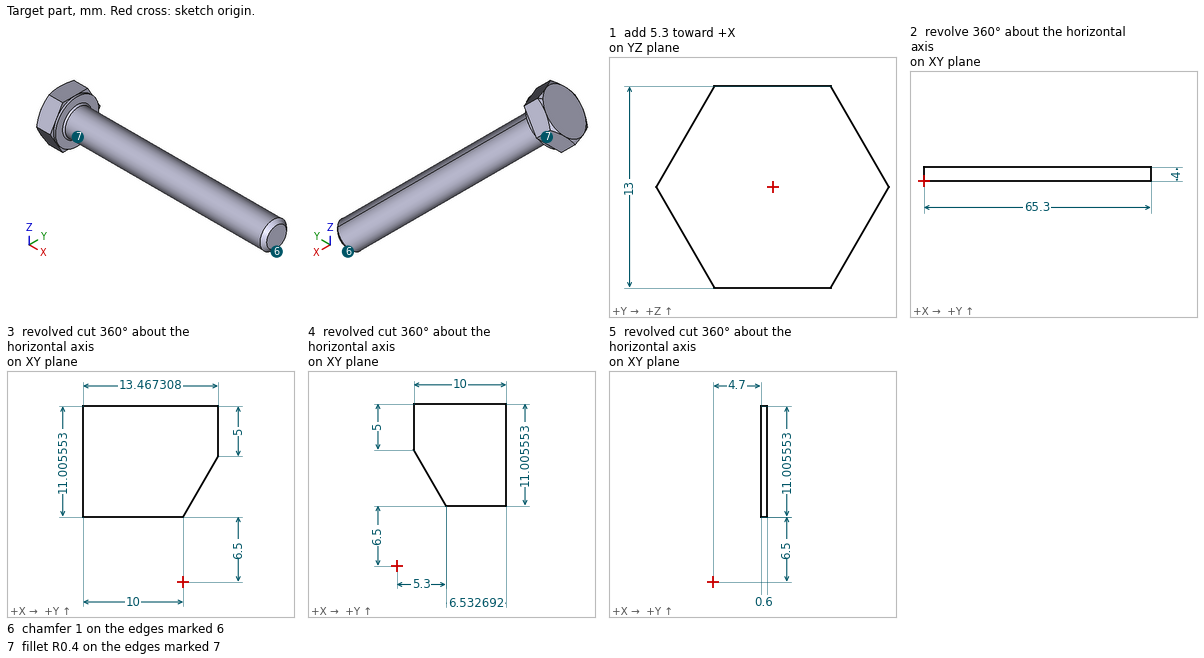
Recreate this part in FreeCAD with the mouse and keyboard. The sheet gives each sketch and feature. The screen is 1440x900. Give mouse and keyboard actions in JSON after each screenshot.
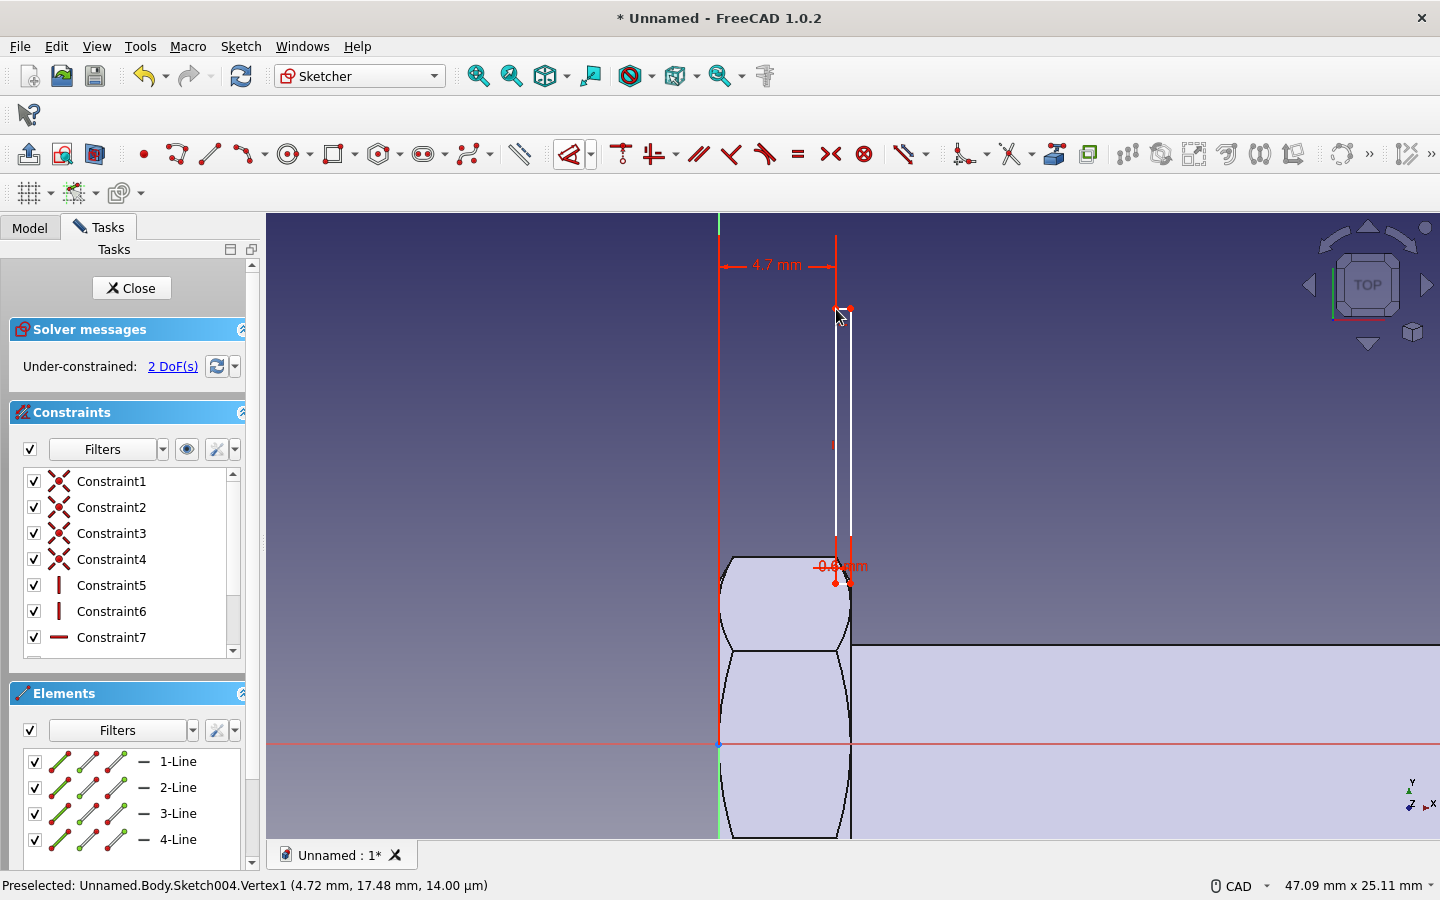
{"action": "left_click", "coordinate": [836, 584]}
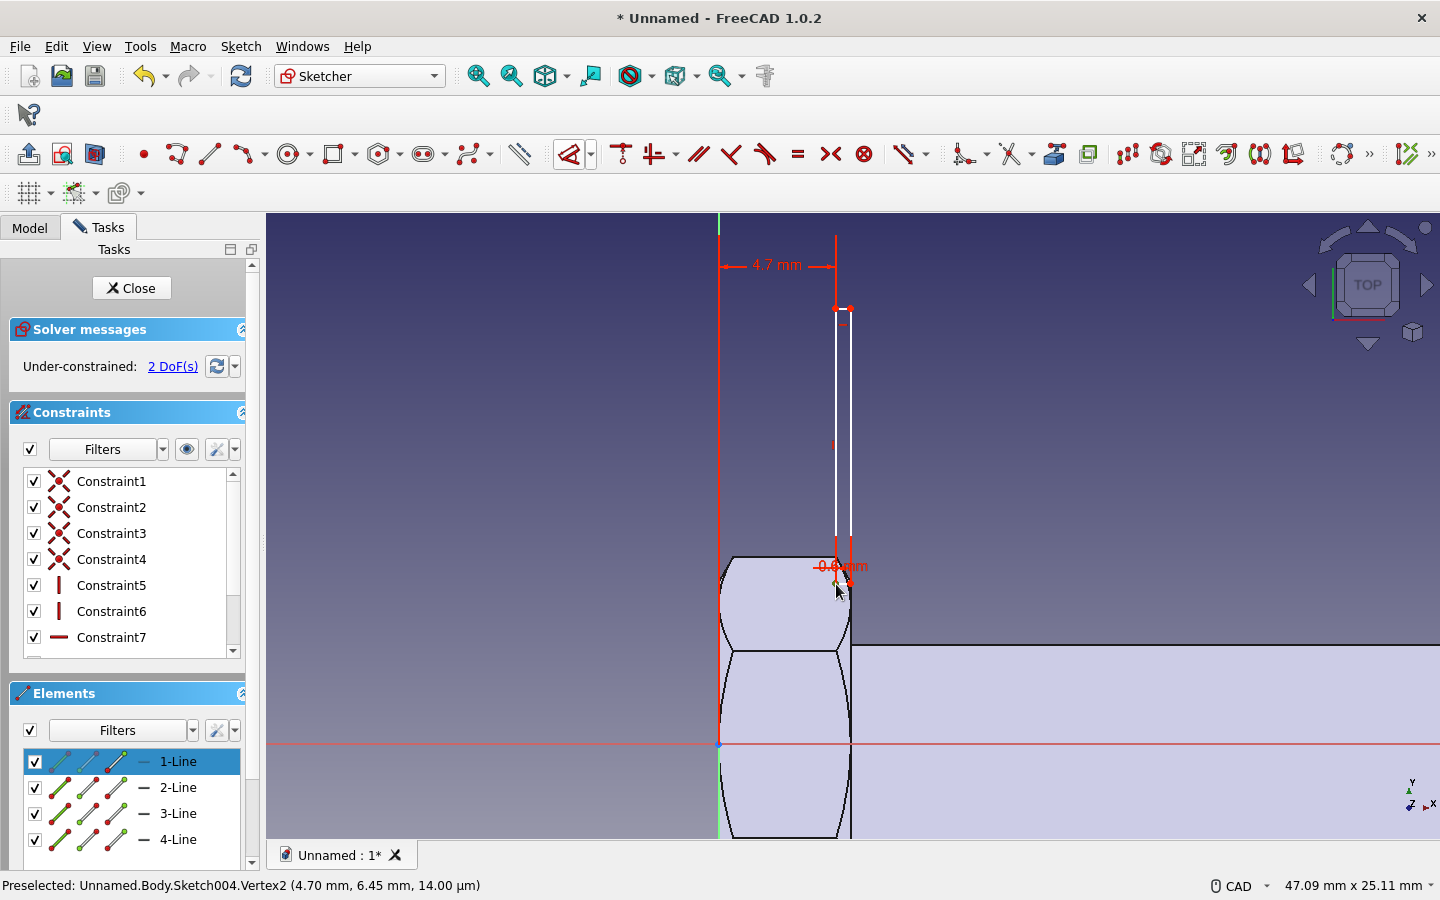
{"action": "key", "text": "i"}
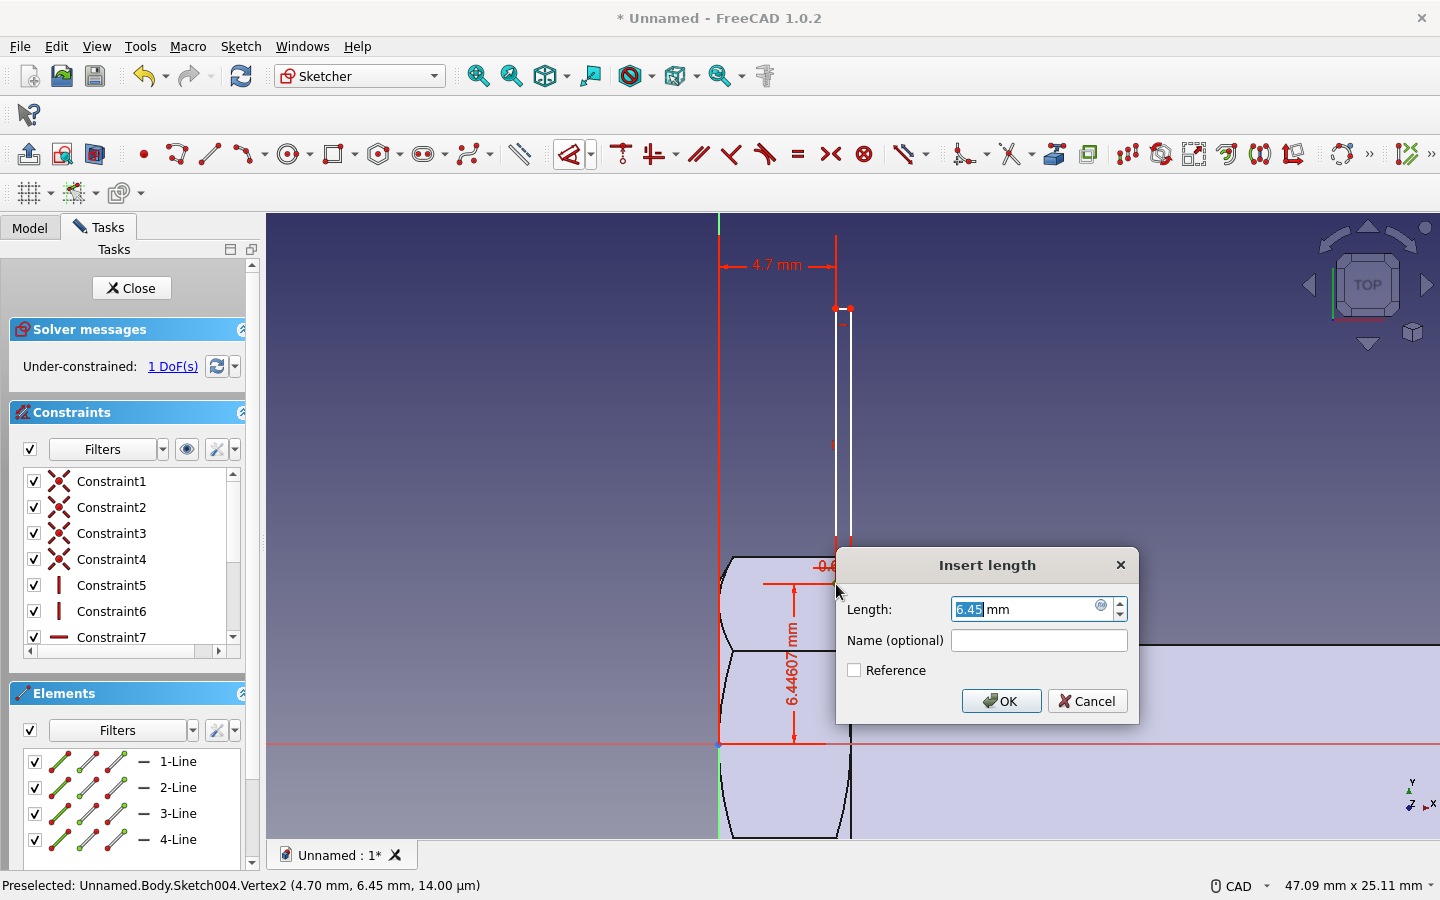
{"action": "type", "text": "6.5"}
{"action": "key", "text": "Return"}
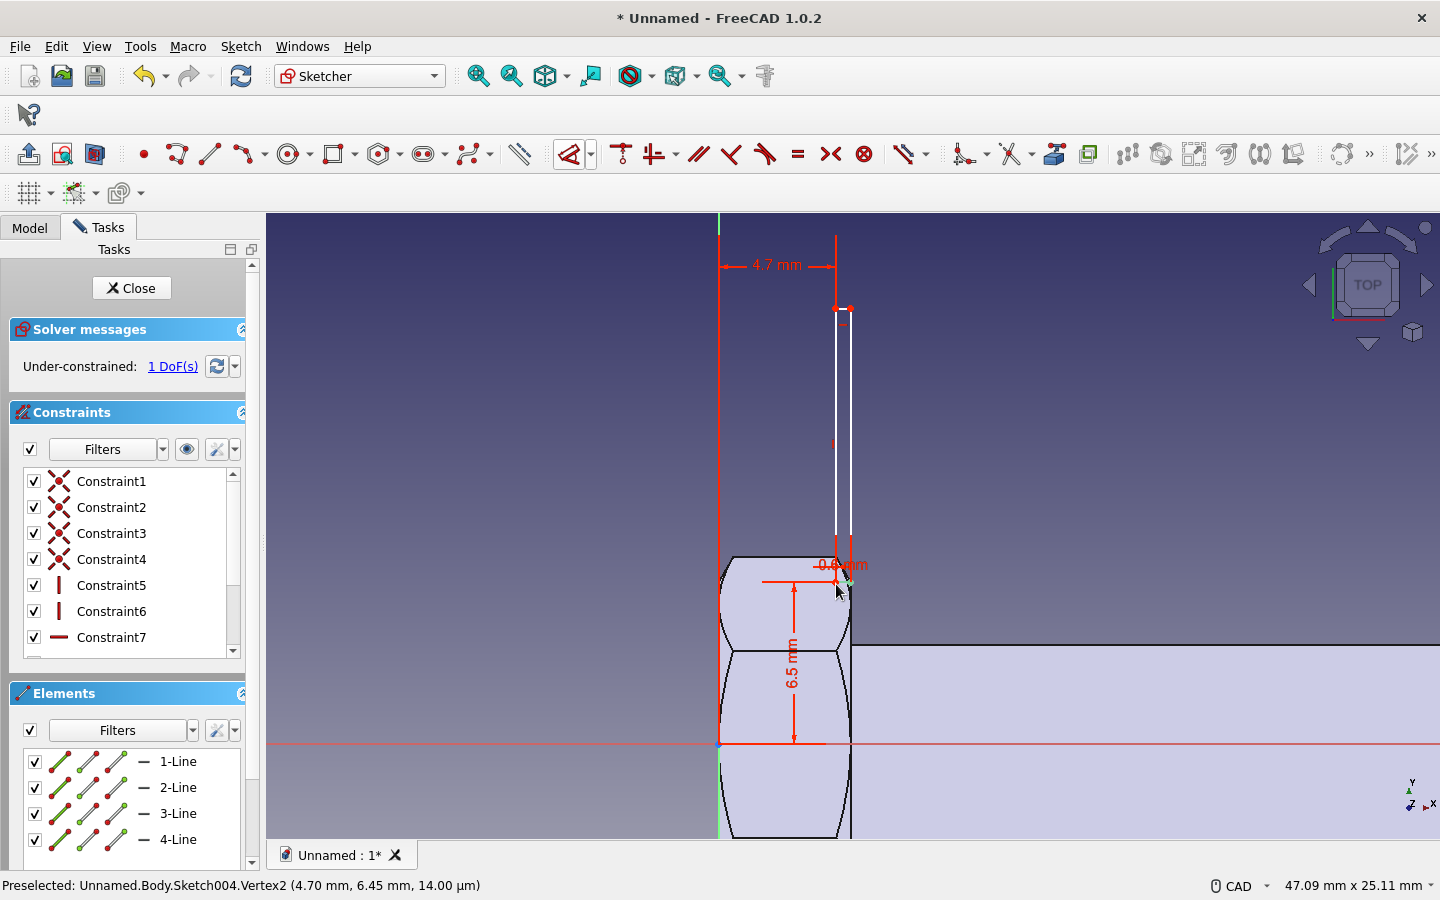
{"action": "left_click", "coordinate": [836, 391]}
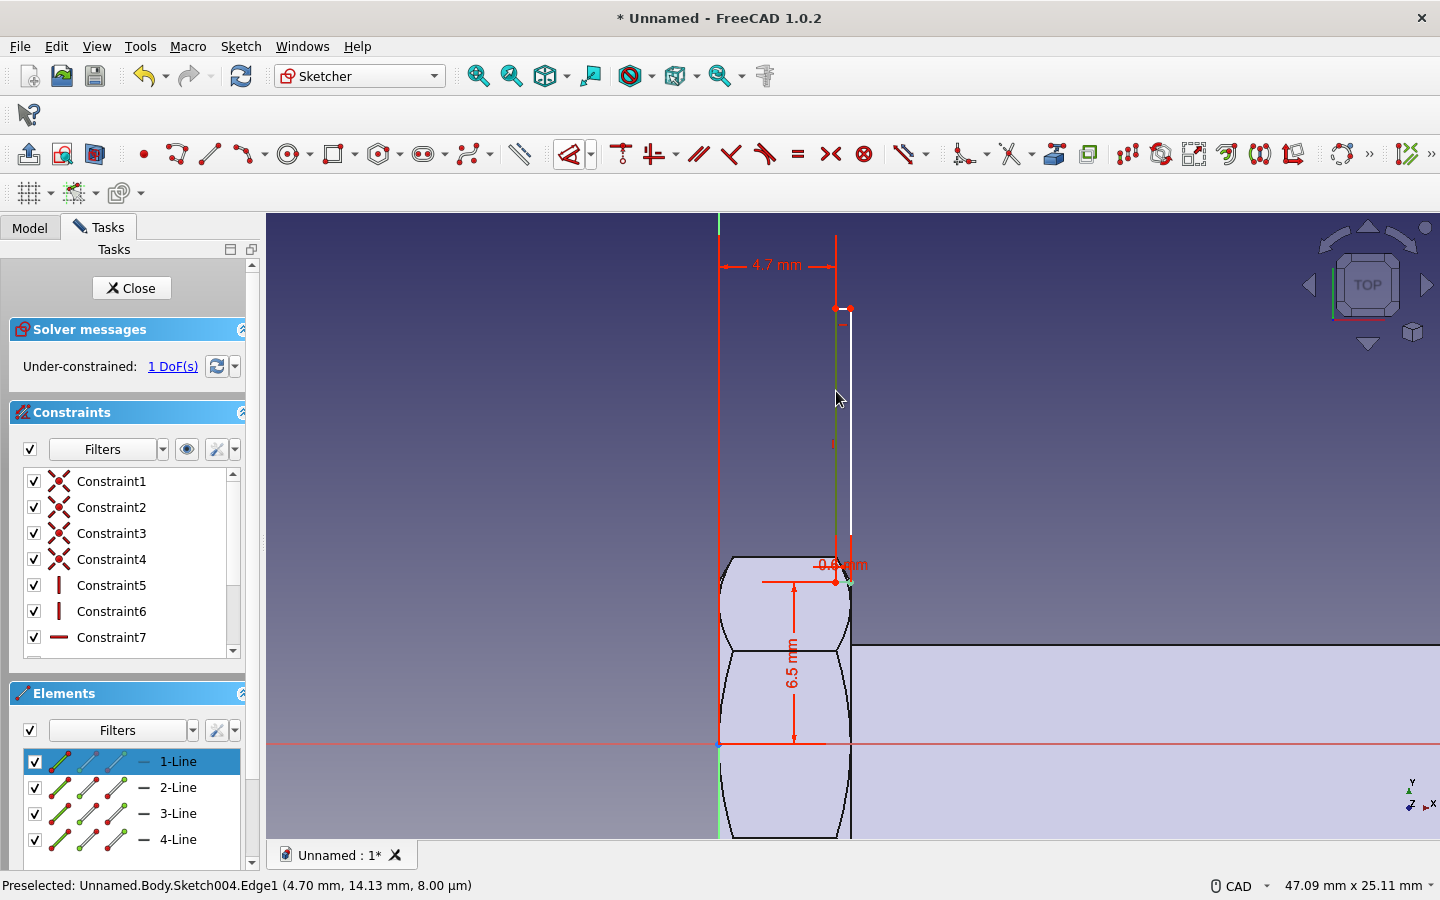
{"action": "left_click", "coordinate": [590, 154]}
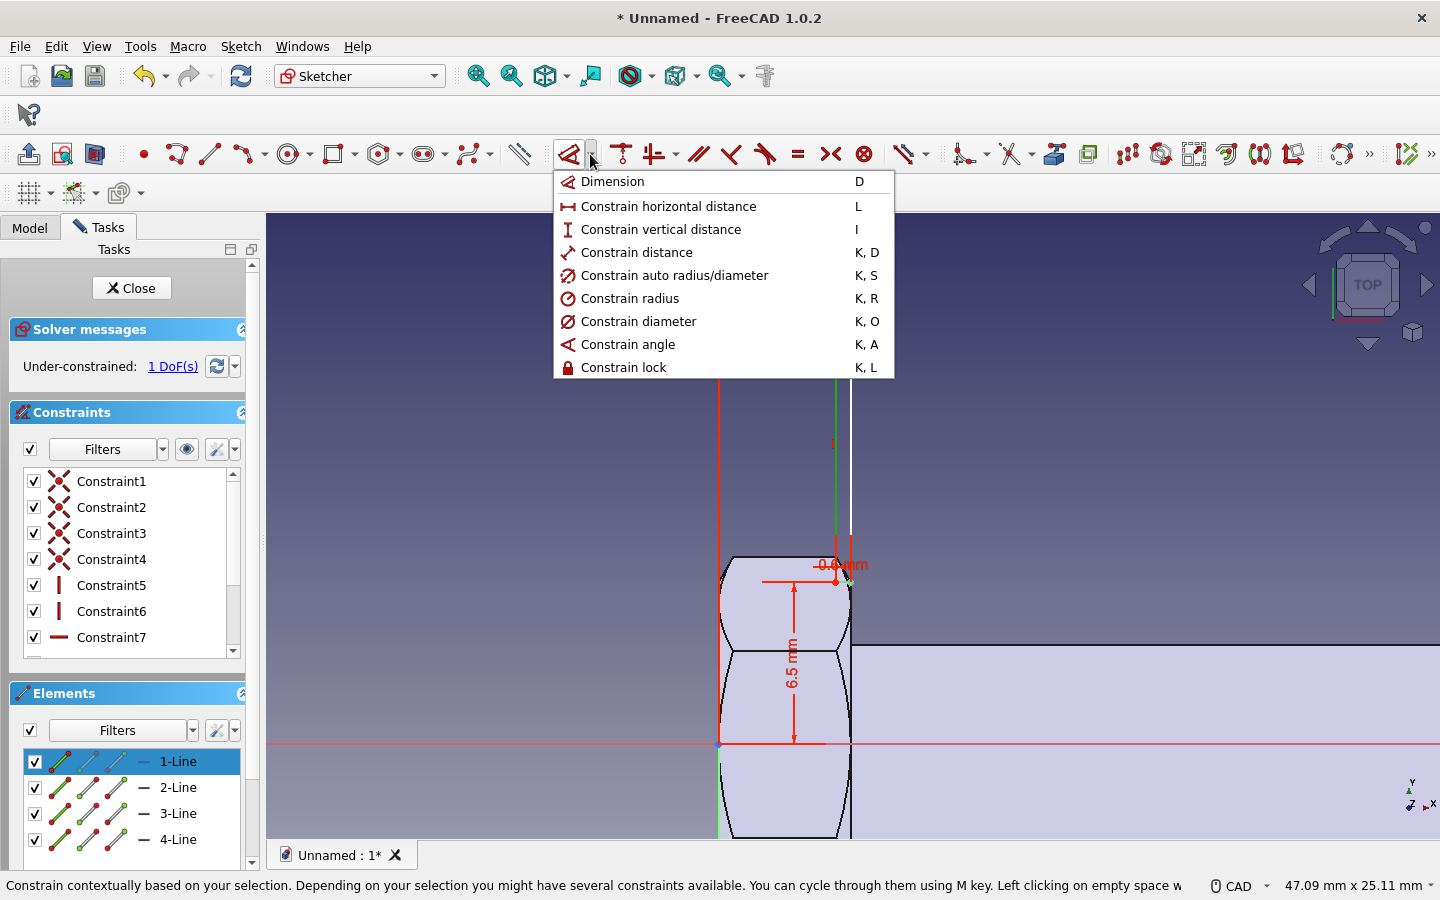
{"action": "left_click", "coordinate": [724, 230]}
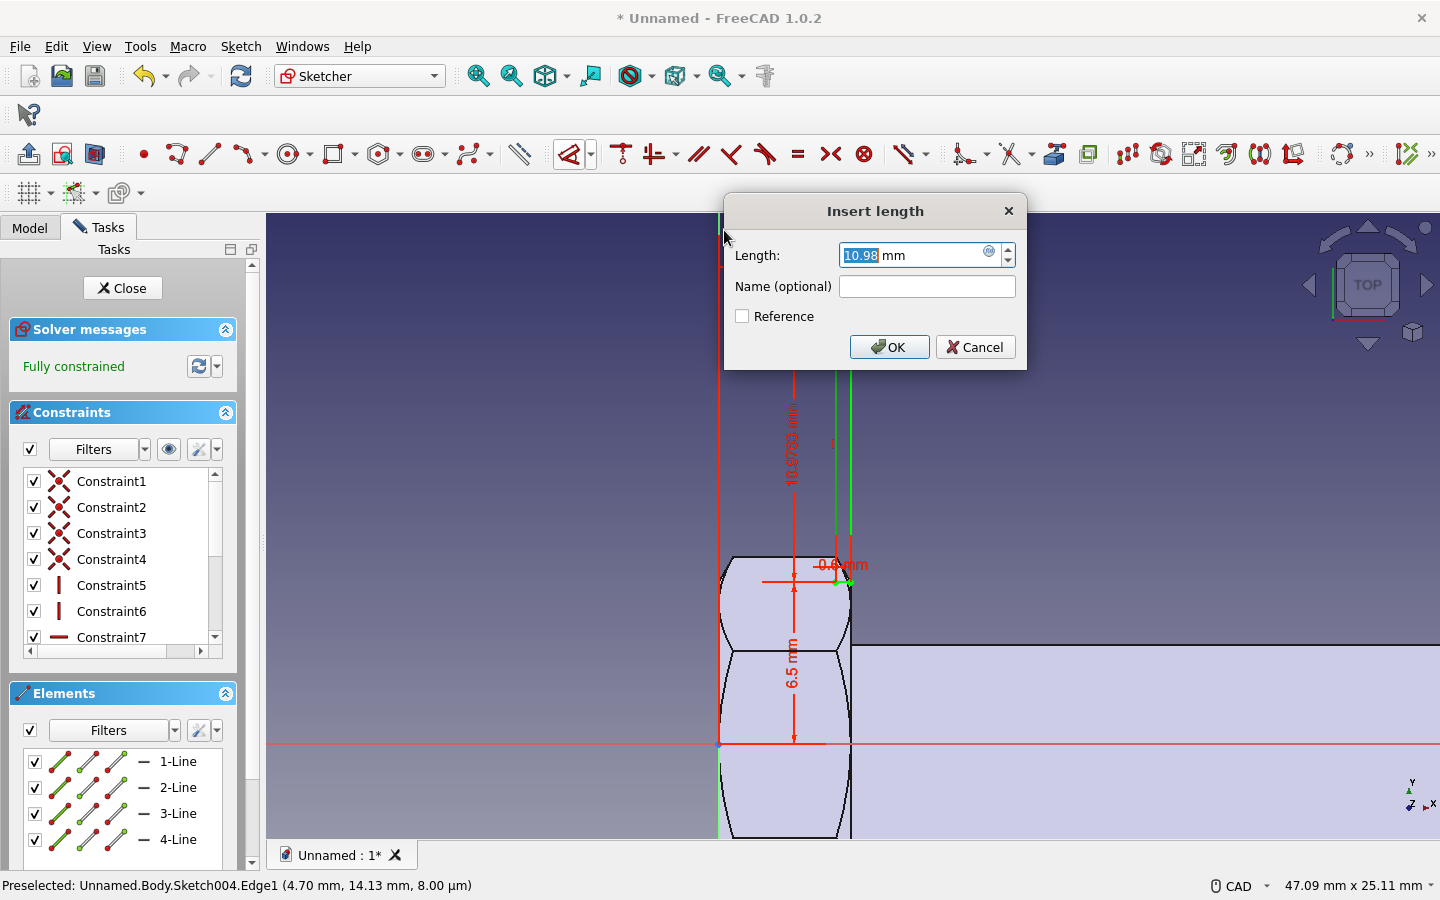
{"action": "type", "text": "11.005553"}
{"action": "key", "text": "Return"}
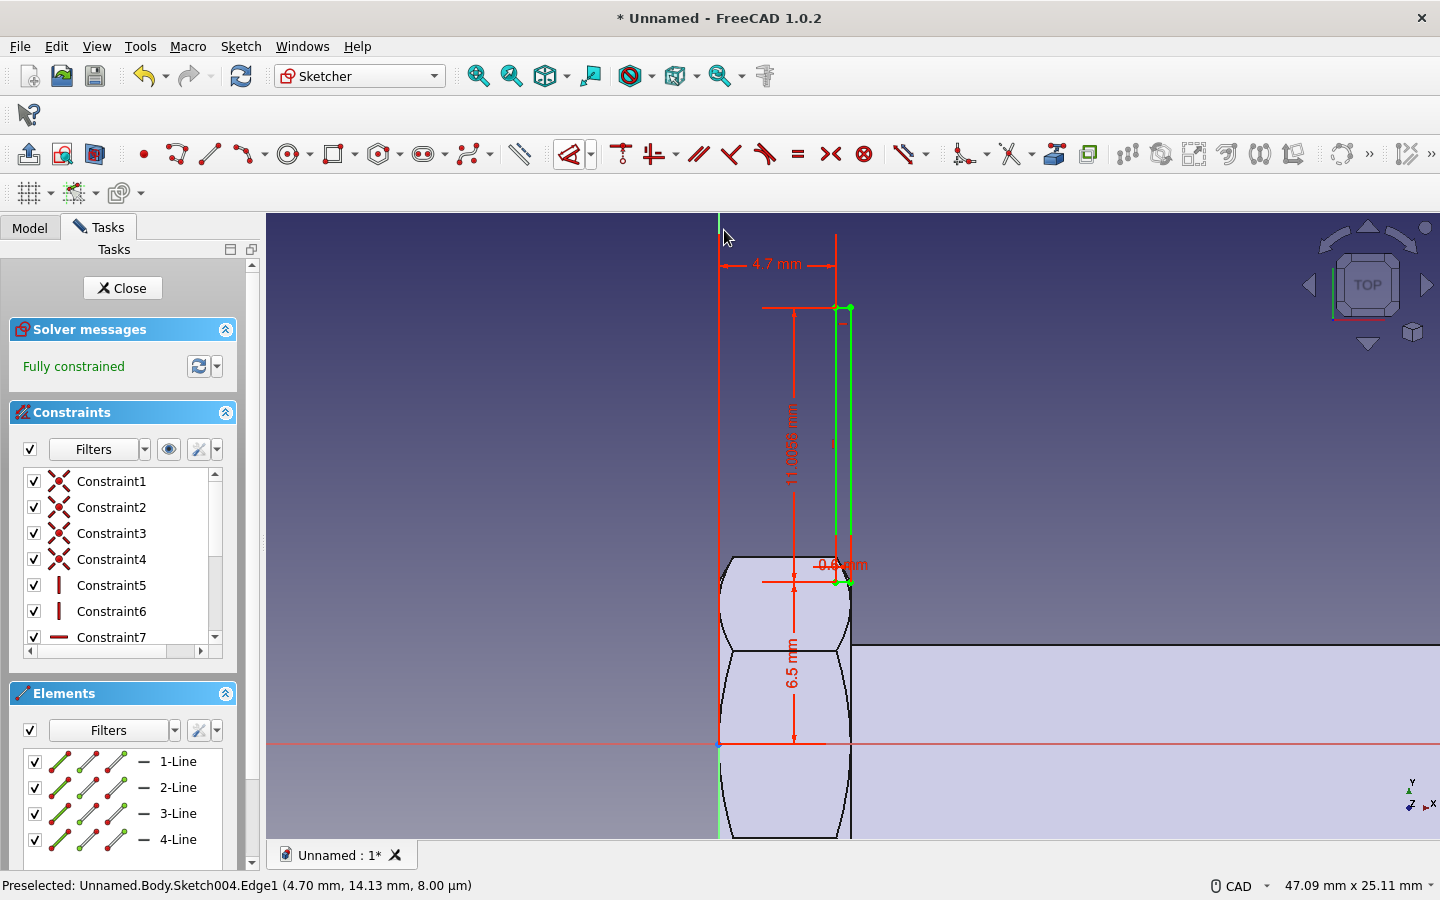
{"action": "left_click", "coordinate": [123, 288]}